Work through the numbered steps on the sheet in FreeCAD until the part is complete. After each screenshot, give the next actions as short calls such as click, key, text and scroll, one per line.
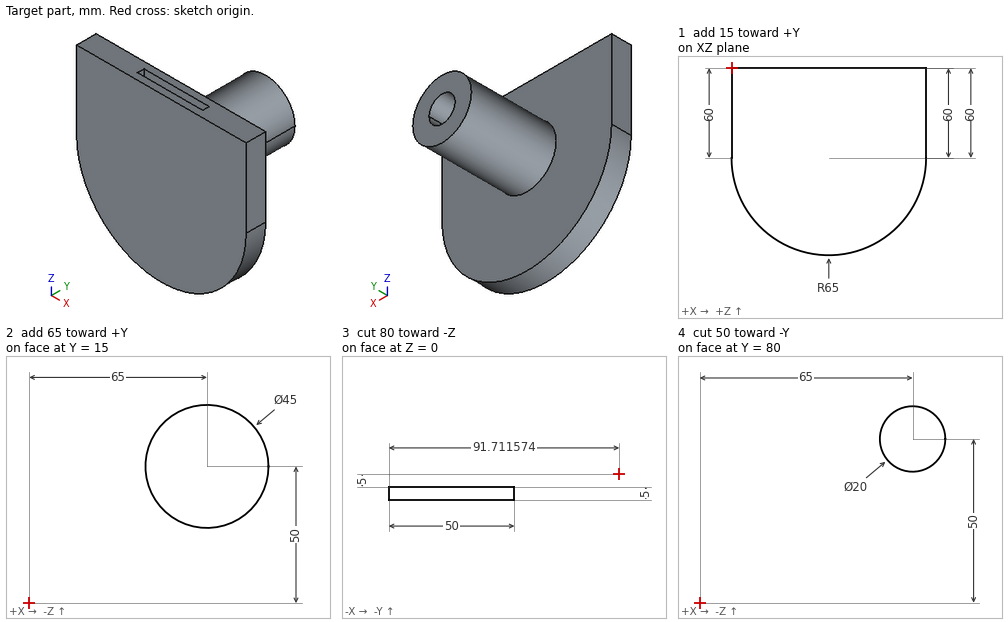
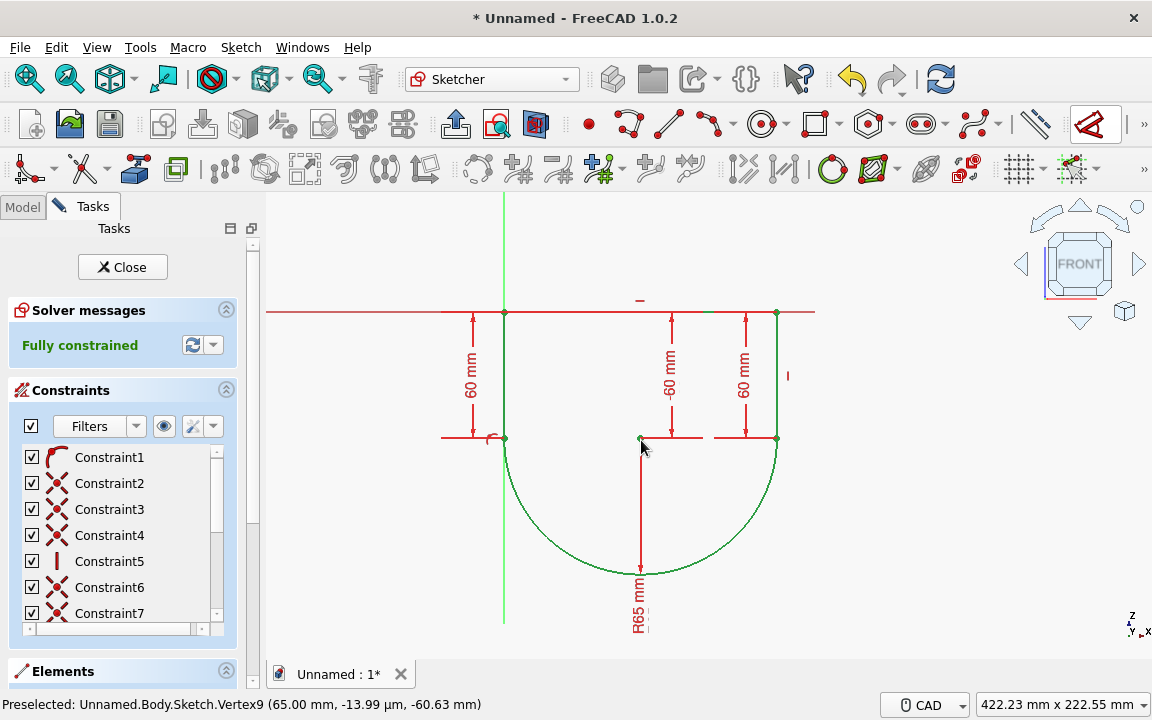
click(123, 267)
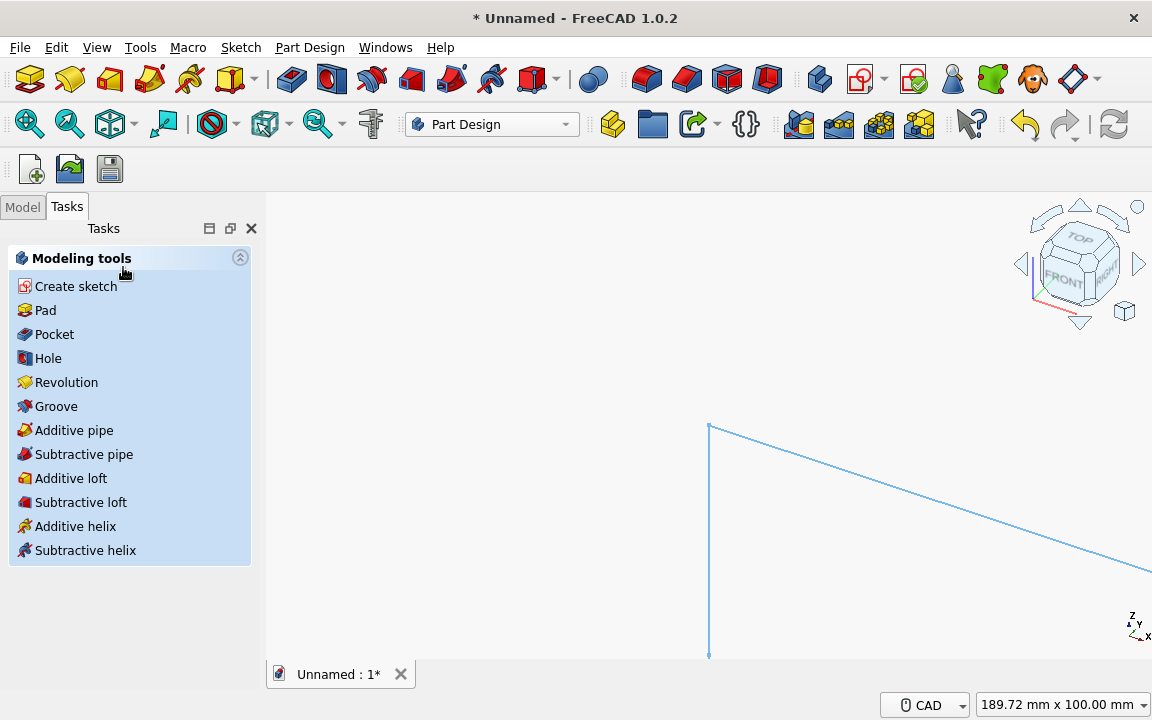
click(30, 80)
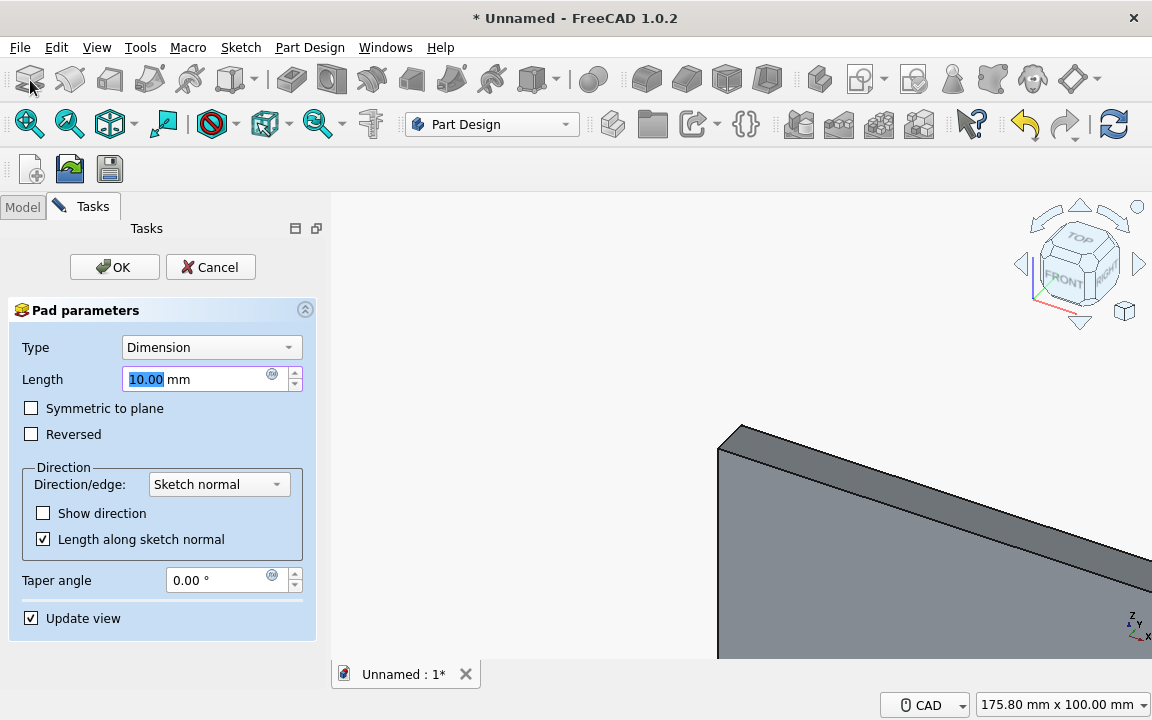
text(15)
key(Tab)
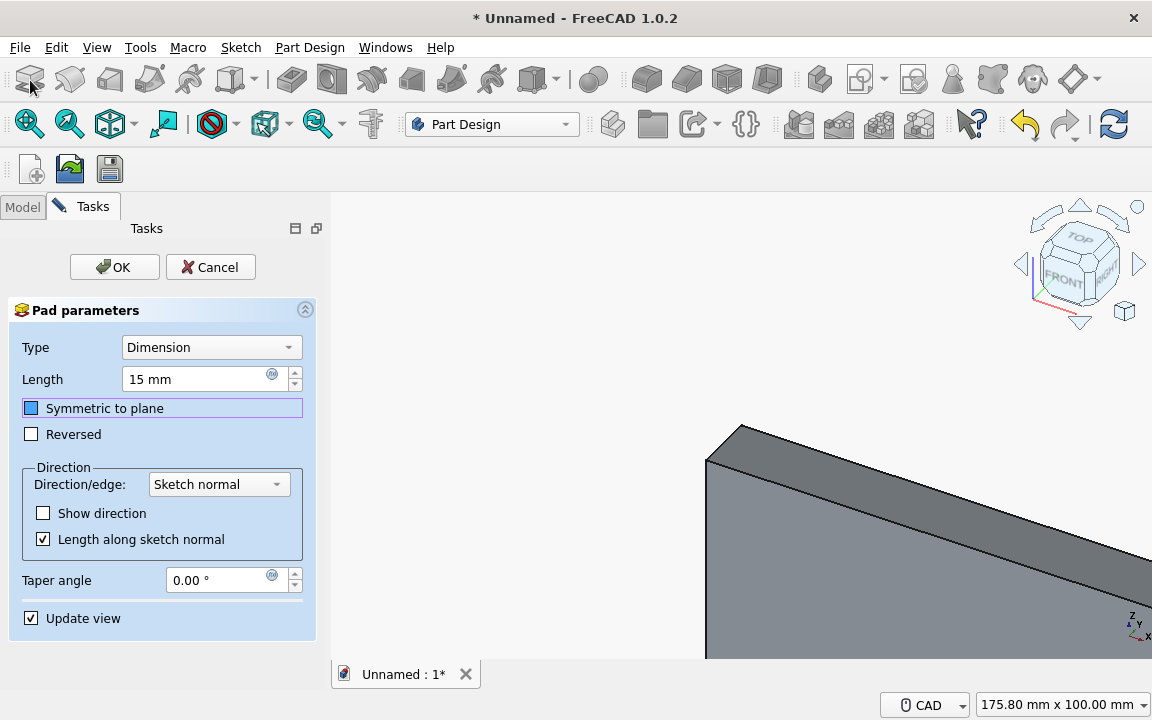
click(30, 434)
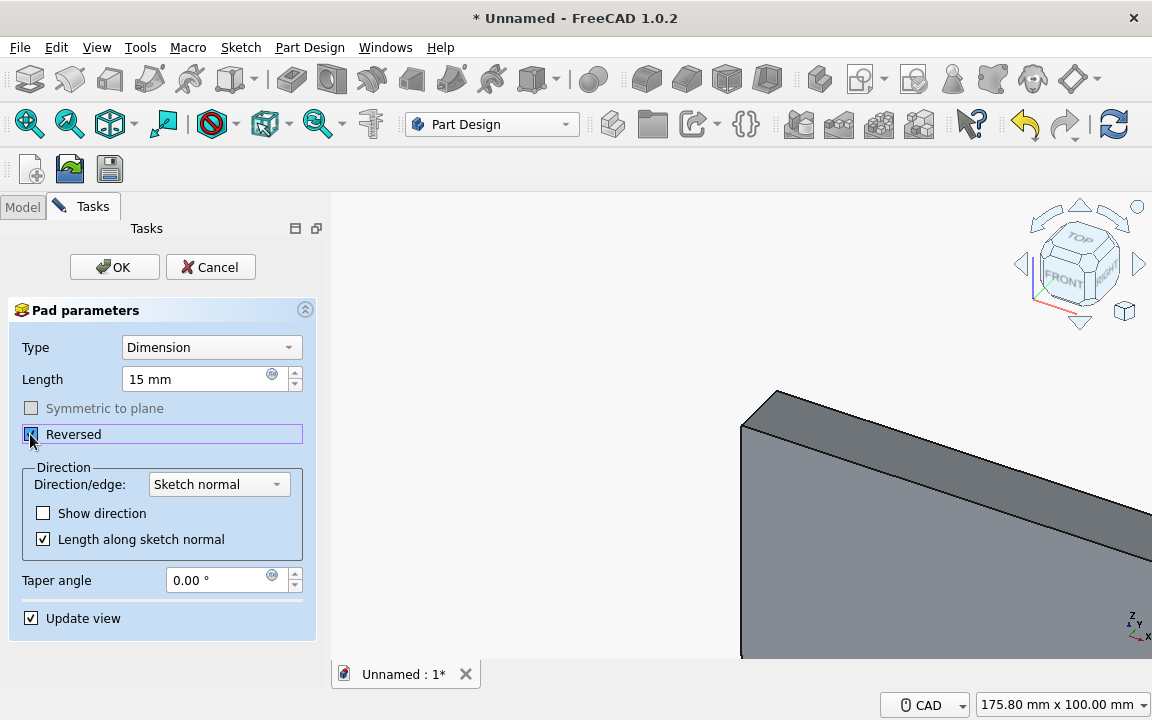
click(115, 267)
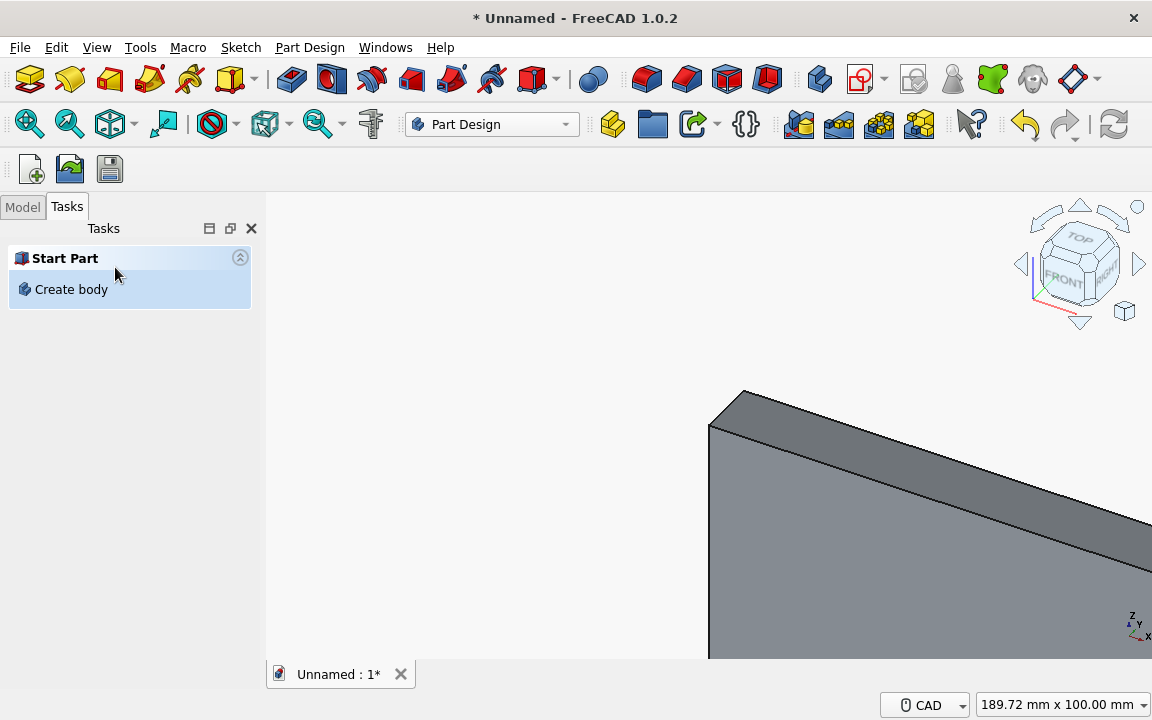
click(30, 124)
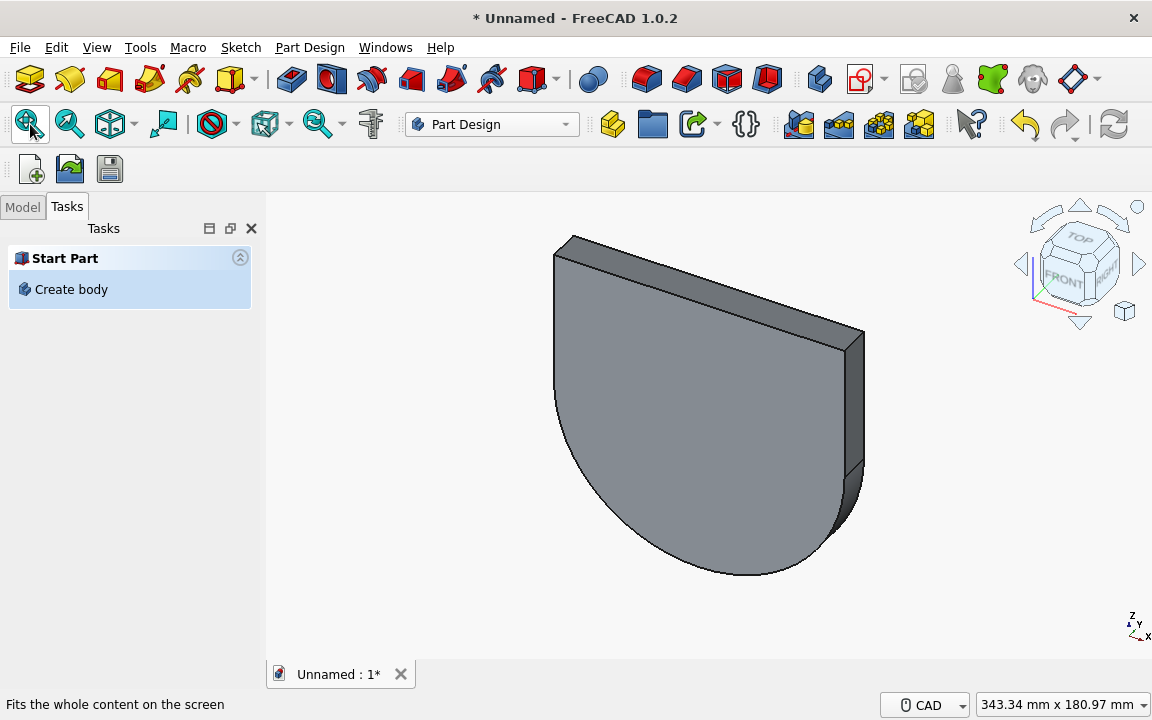
key(4)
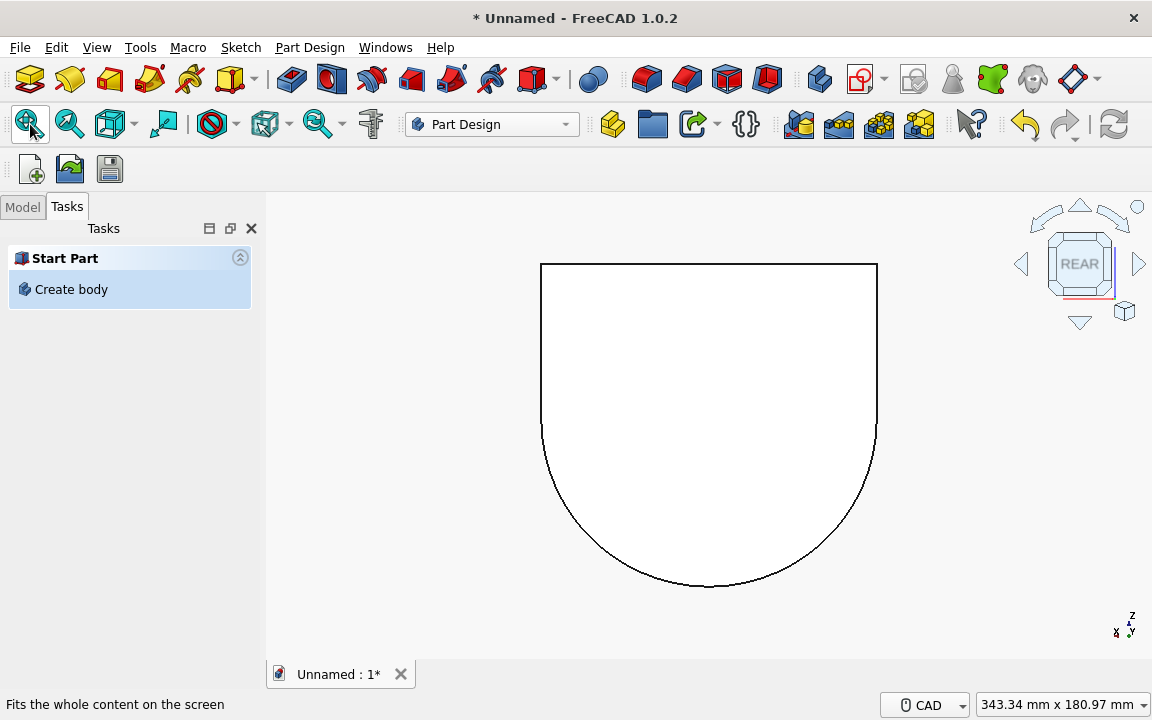
click(709, 424)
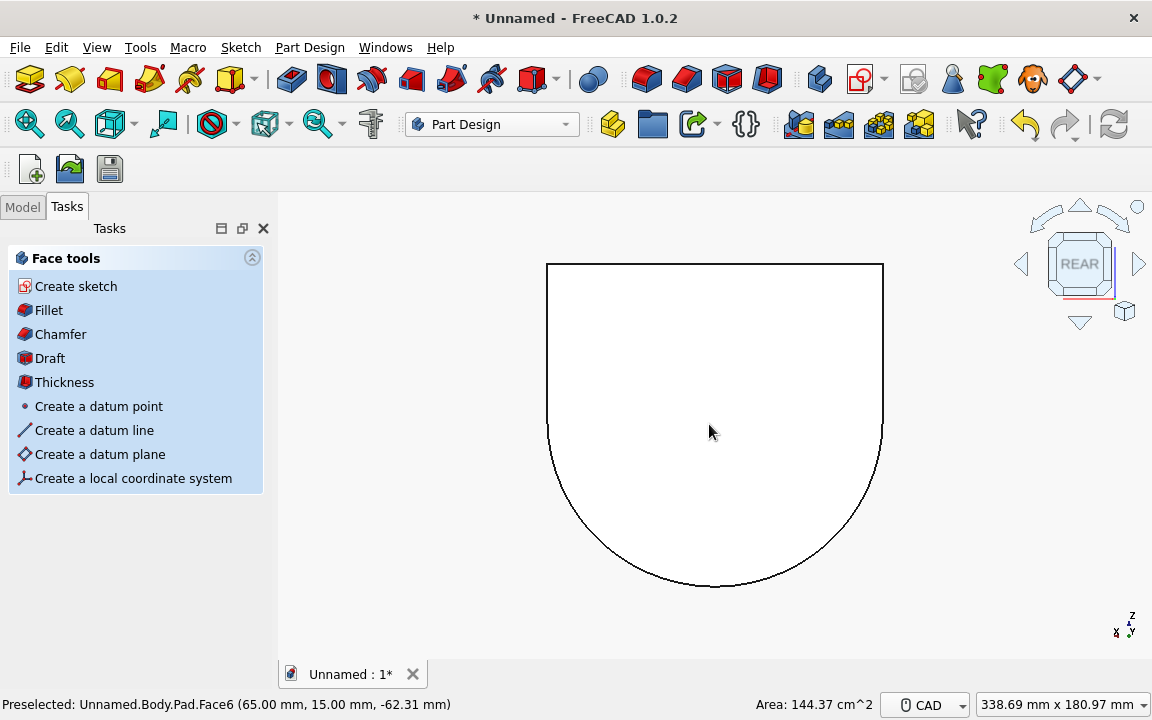
click(860, 80)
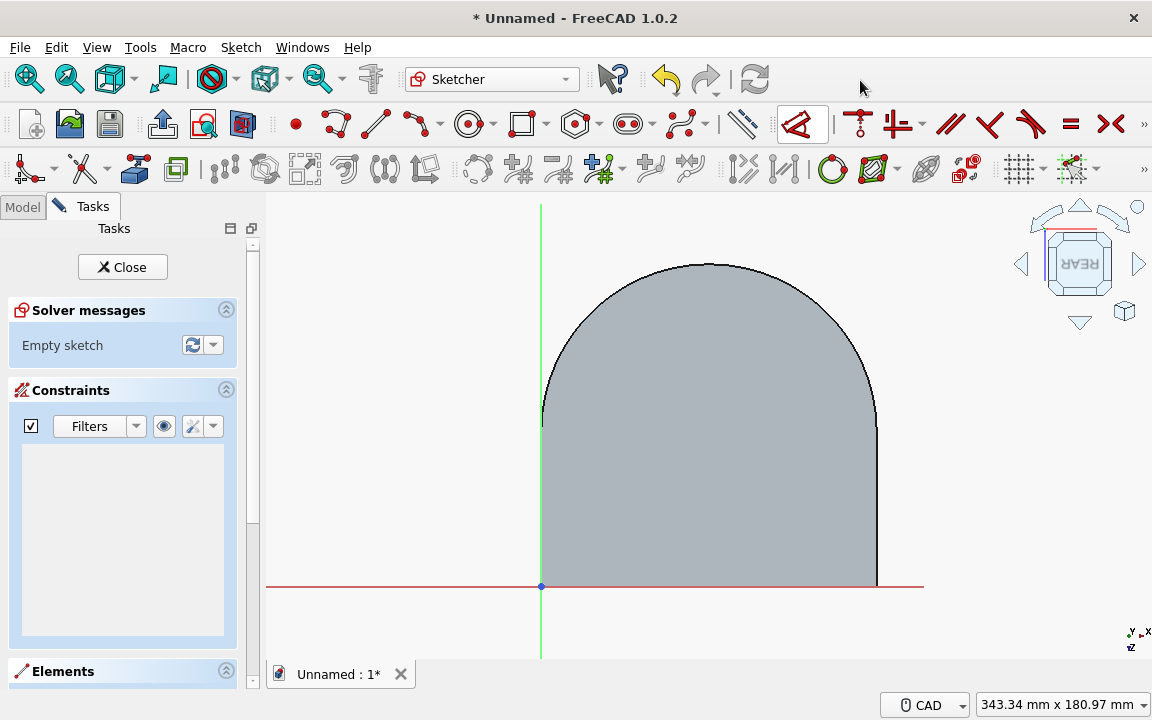
scroll(682, 631, up, 2)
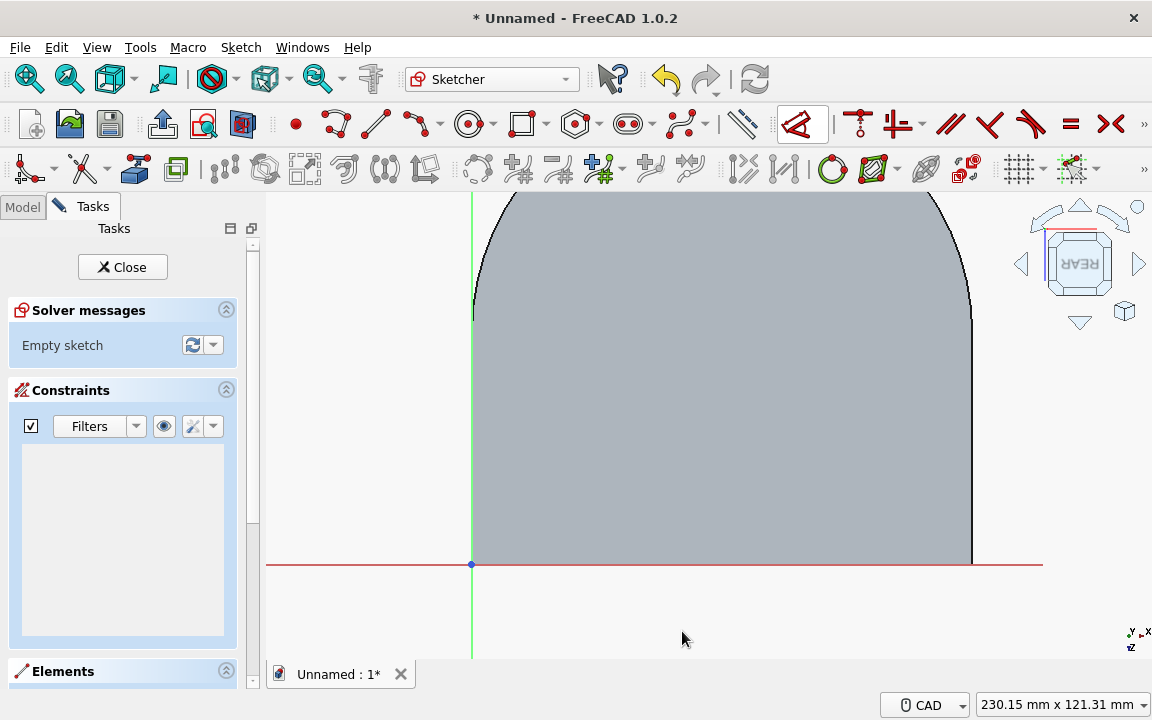
click(470, 124)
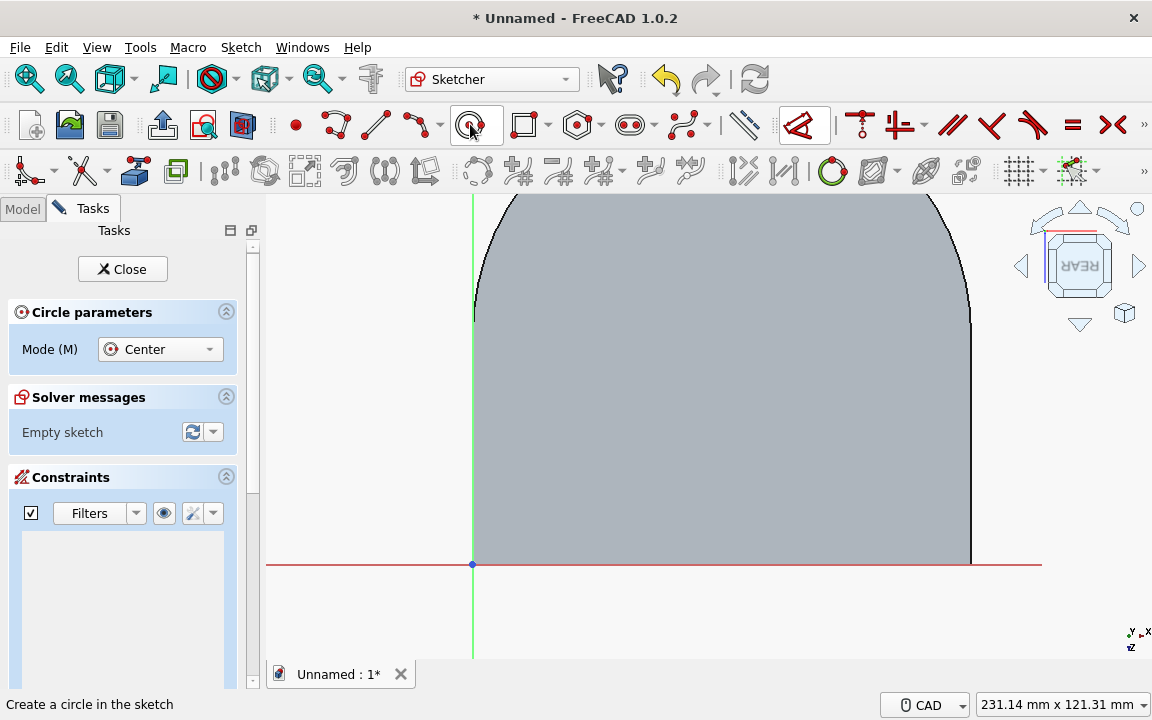
click(722, 373)
move(783, 312)